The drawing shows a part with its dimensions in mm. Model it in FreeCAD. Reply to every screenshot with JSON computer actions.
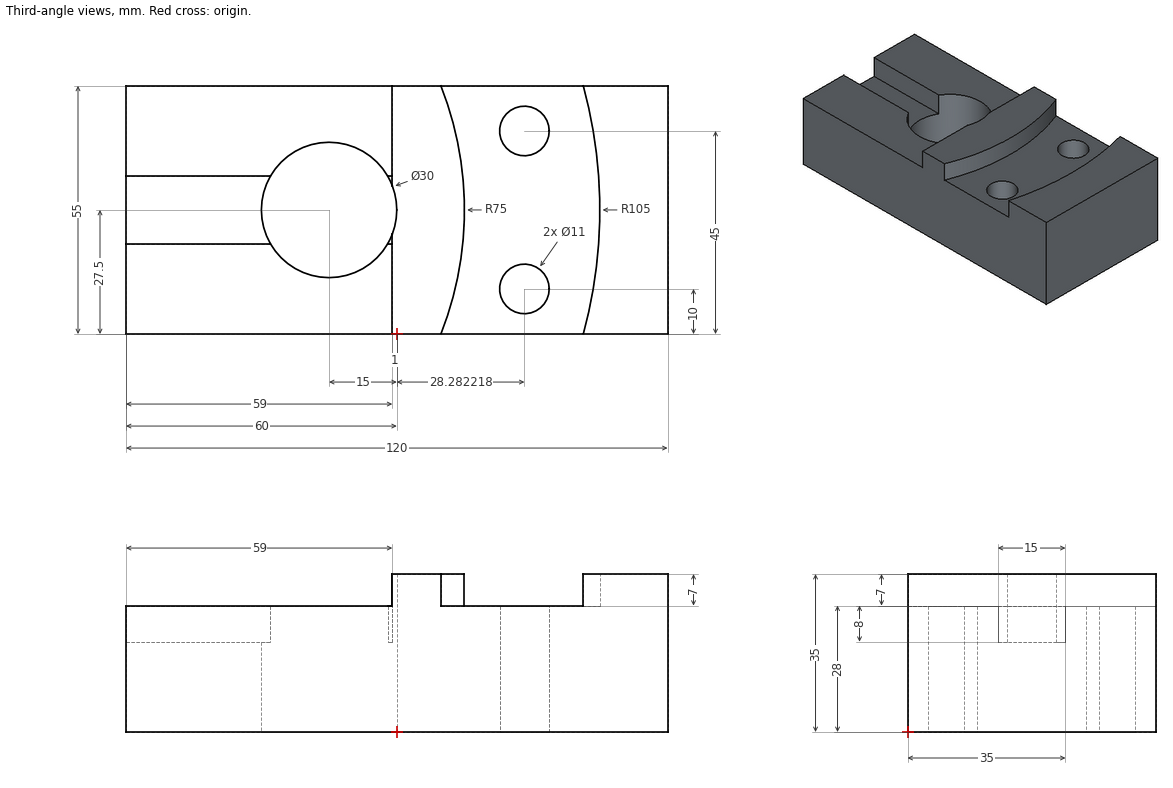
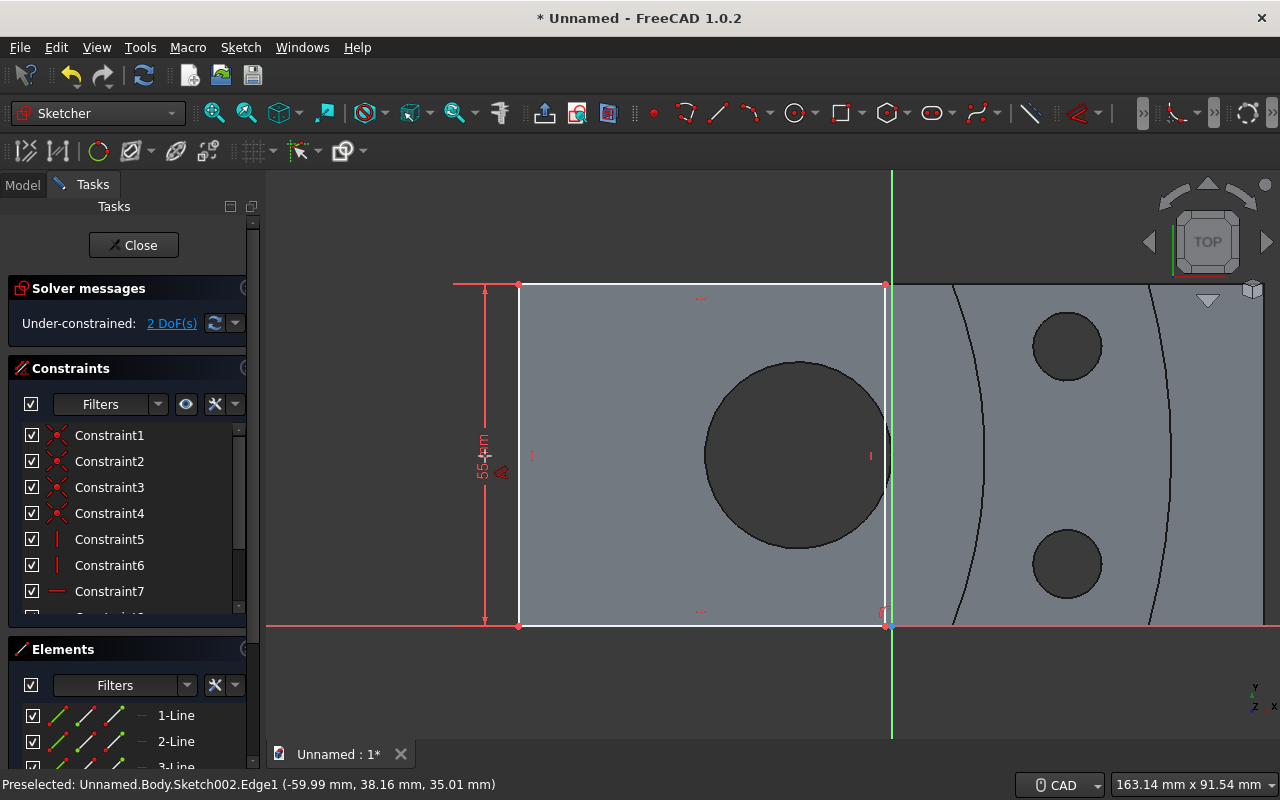
{"action": "left_click", "coordinate": [629, 626]}
{"action": "left_click", "coordinate": [702, 660]}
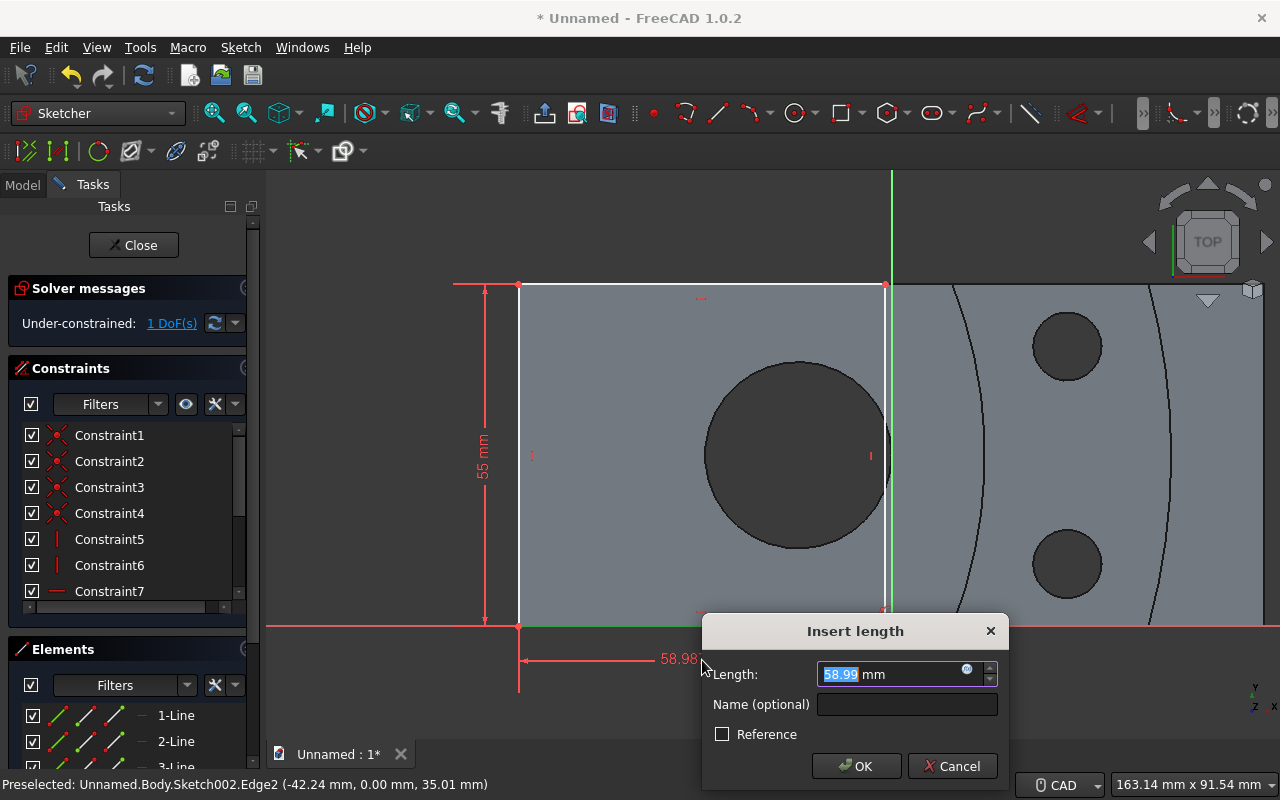
{"action": "type", "text": "59"}
{"action": "key", "text": "Return"}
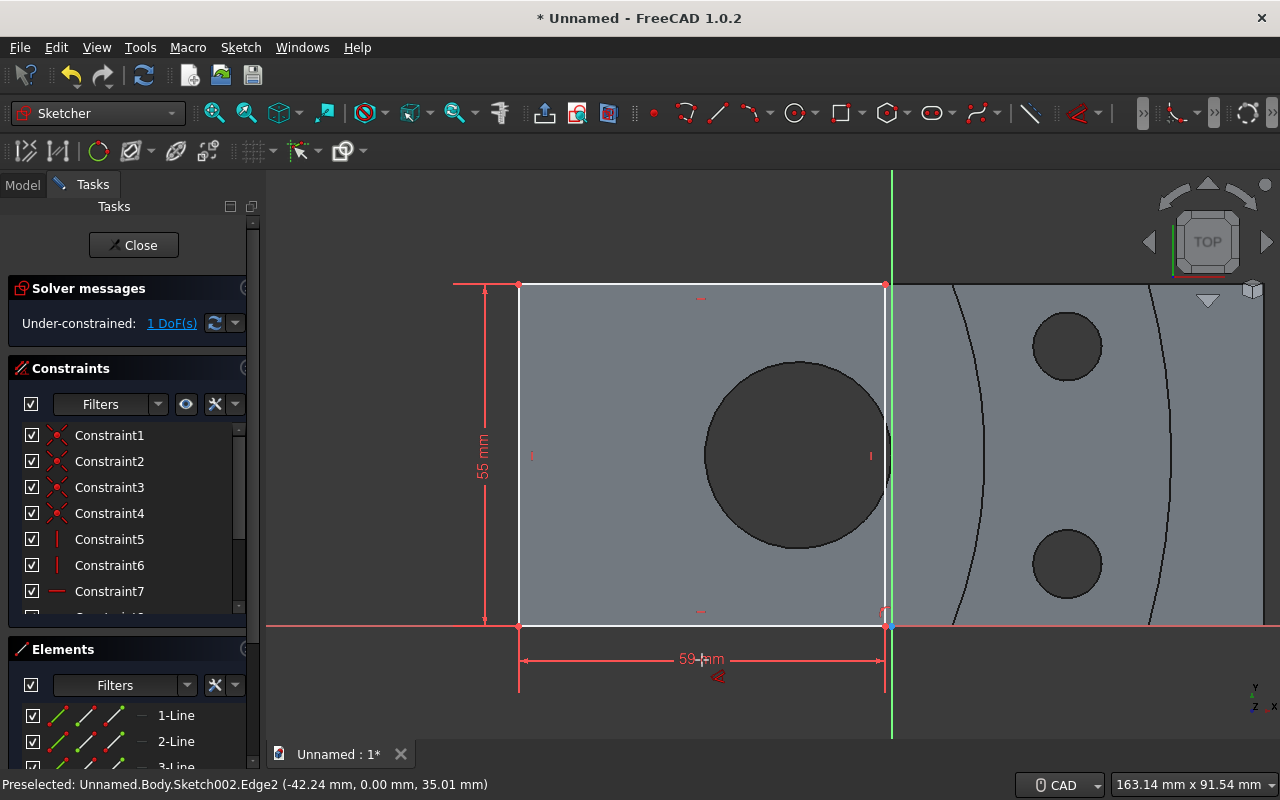
{"action": "scroll", "coordinate": [885, 626], "scroll_direction": "up", "scroll_amount": 10}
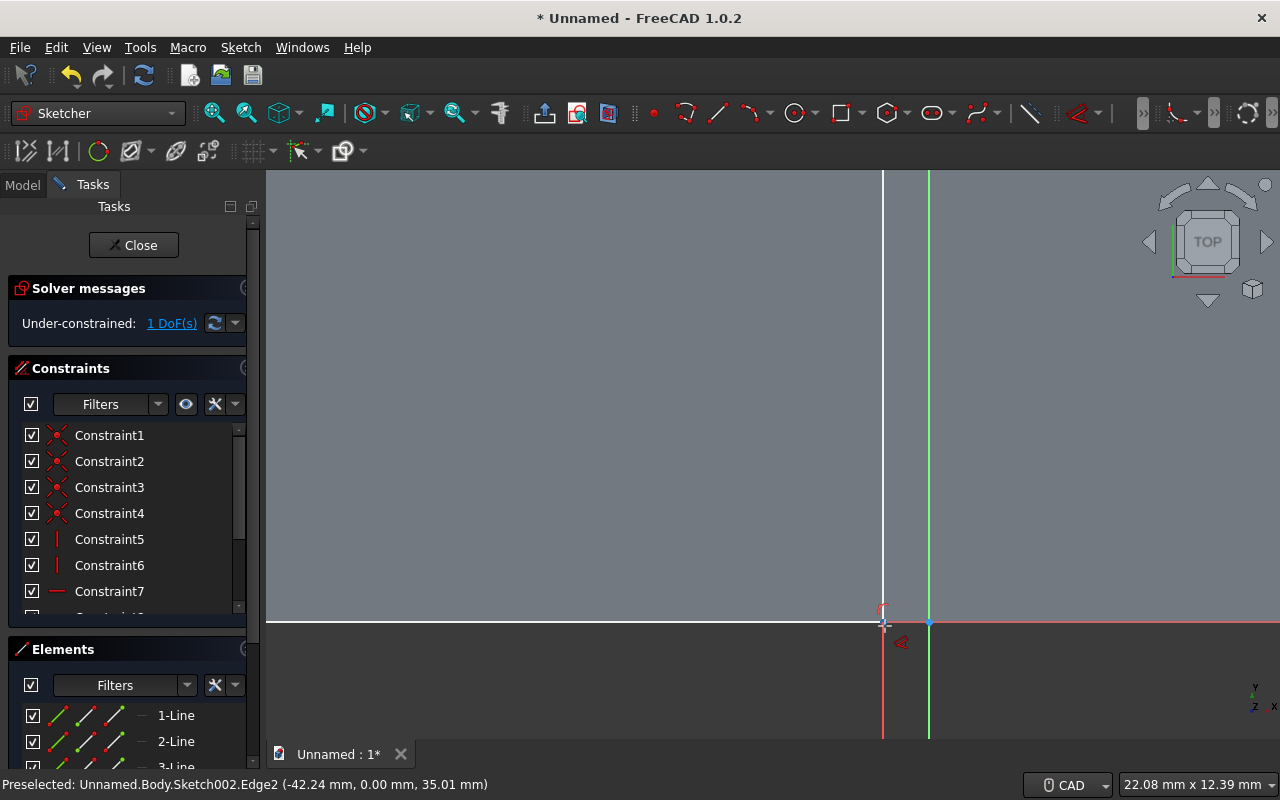
{"action": "left_click", "coordinate": [883, 622]}
{"action": "left_click", "coordinate": [906, 656]}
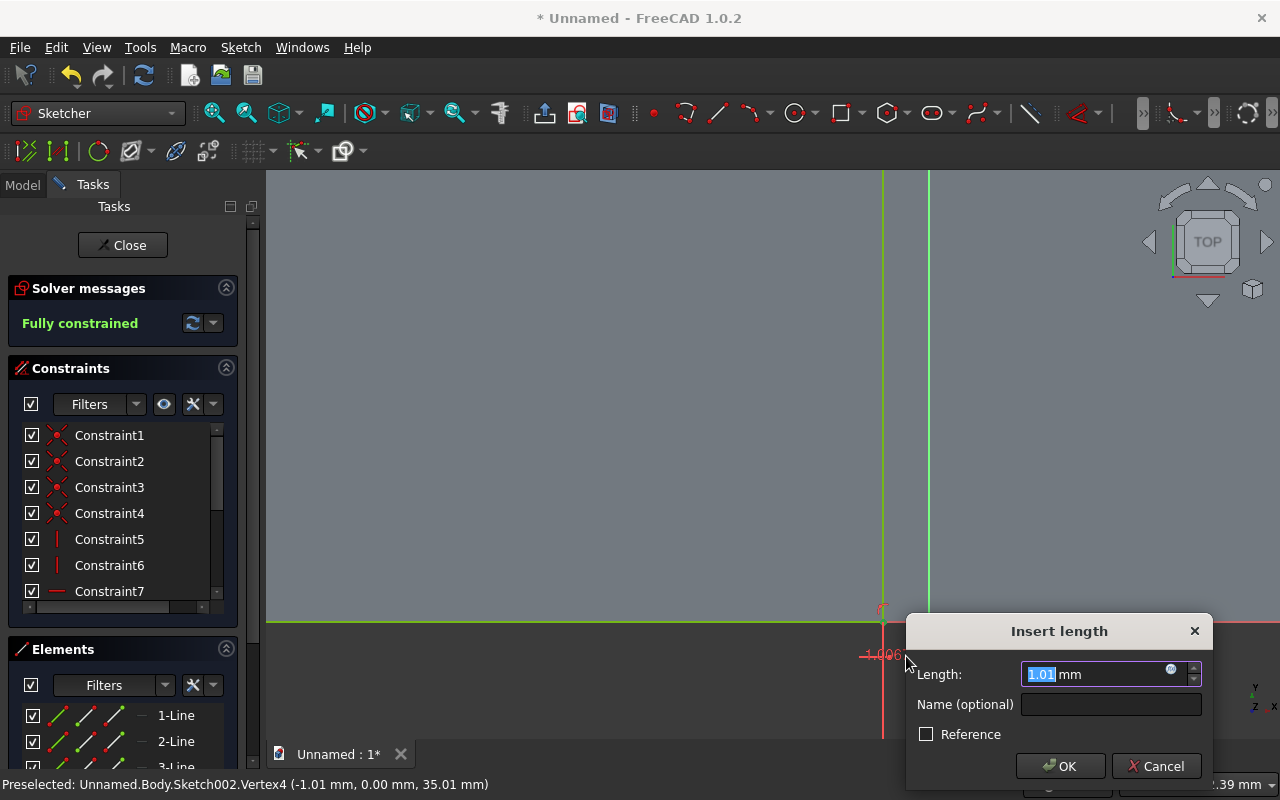
{"action": "type", "text": "1"}
{"action": "key", "text": "Return"}
{"action": "key", "text": "Escape"}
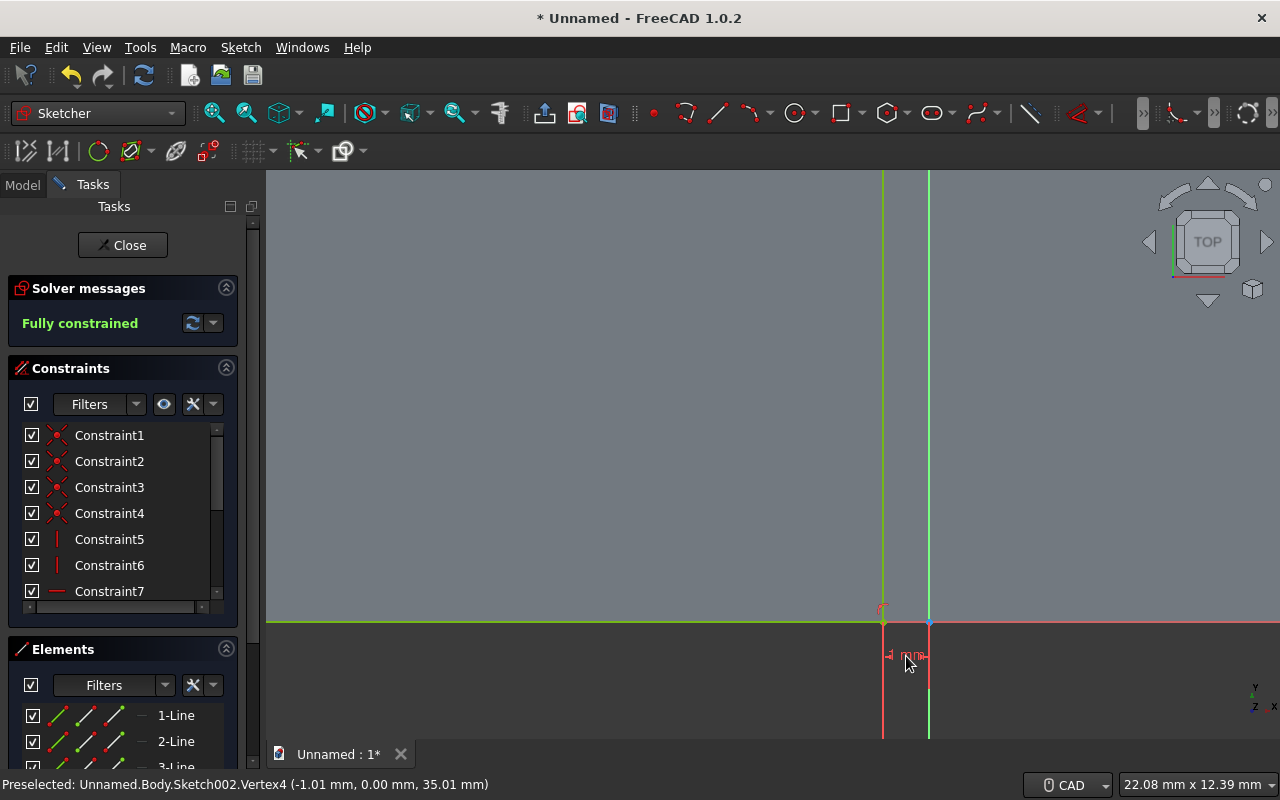
{"action": "left_click", "coordinate": [123, 245]}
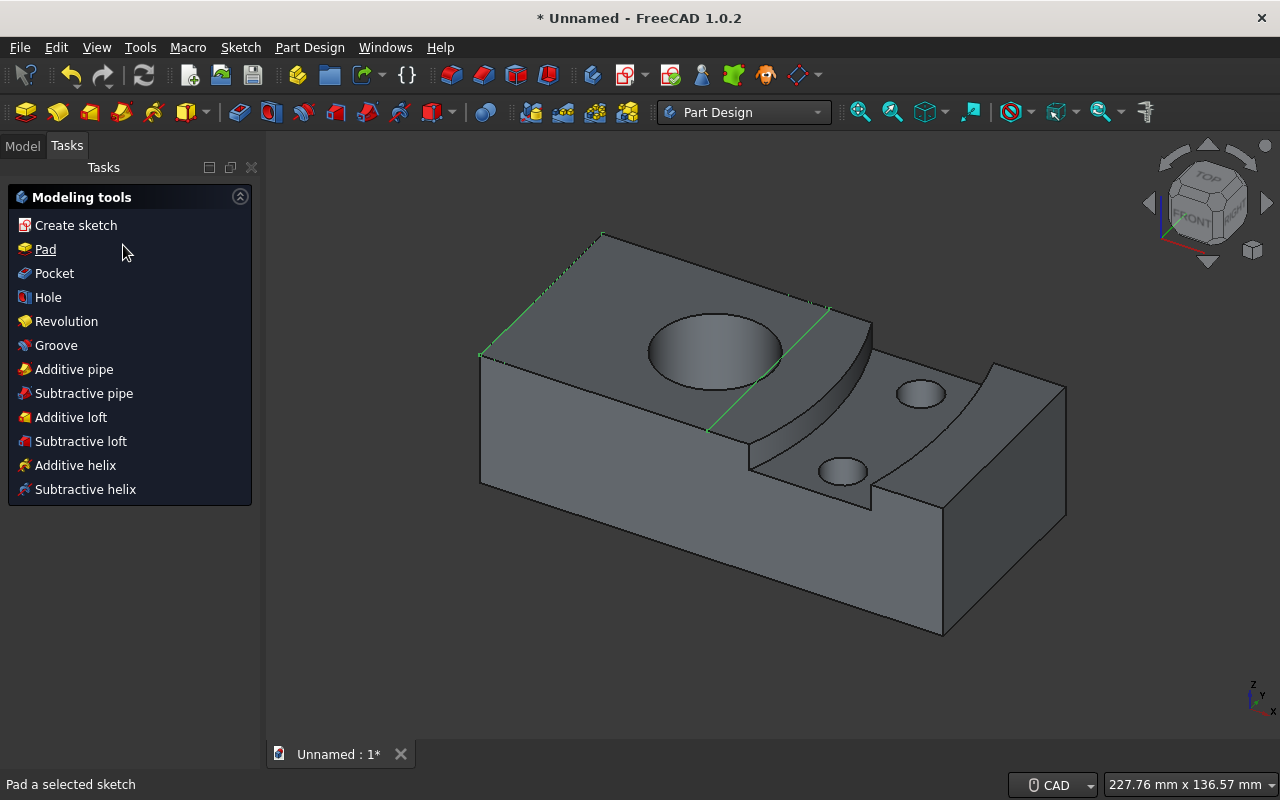
{"action": "left_click", "coordinate": [240, 112]}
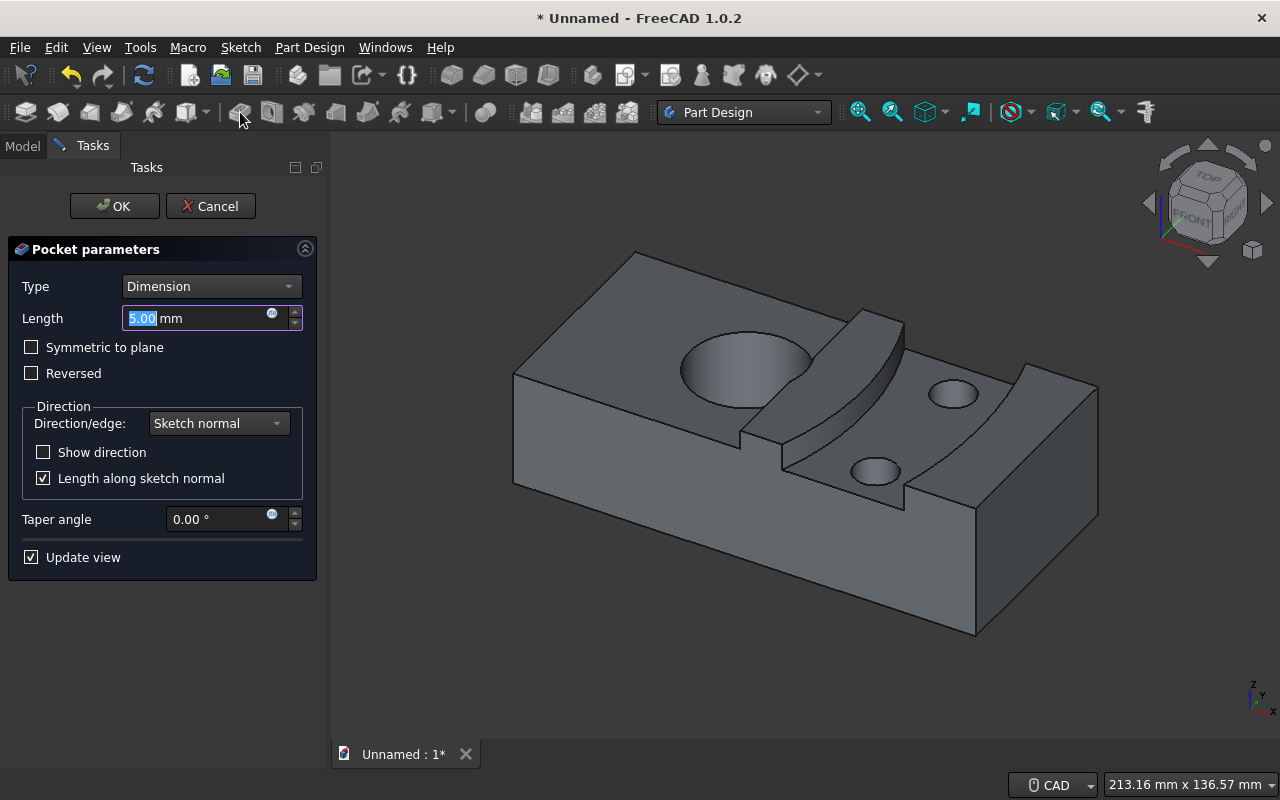
{"action": "type", "text": "7"}
{"action": "key", "text": "Tab"}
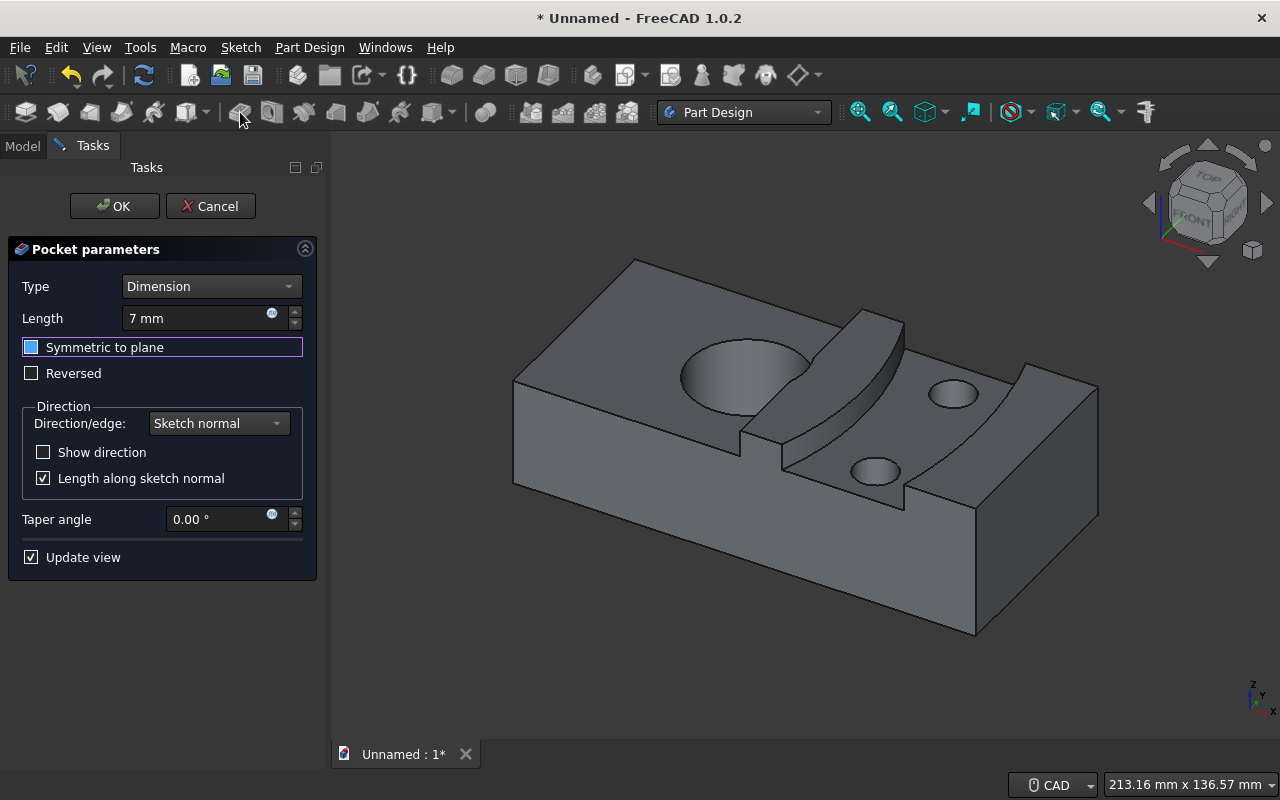
{"action": "left_click", "coordinate": [115, 206]}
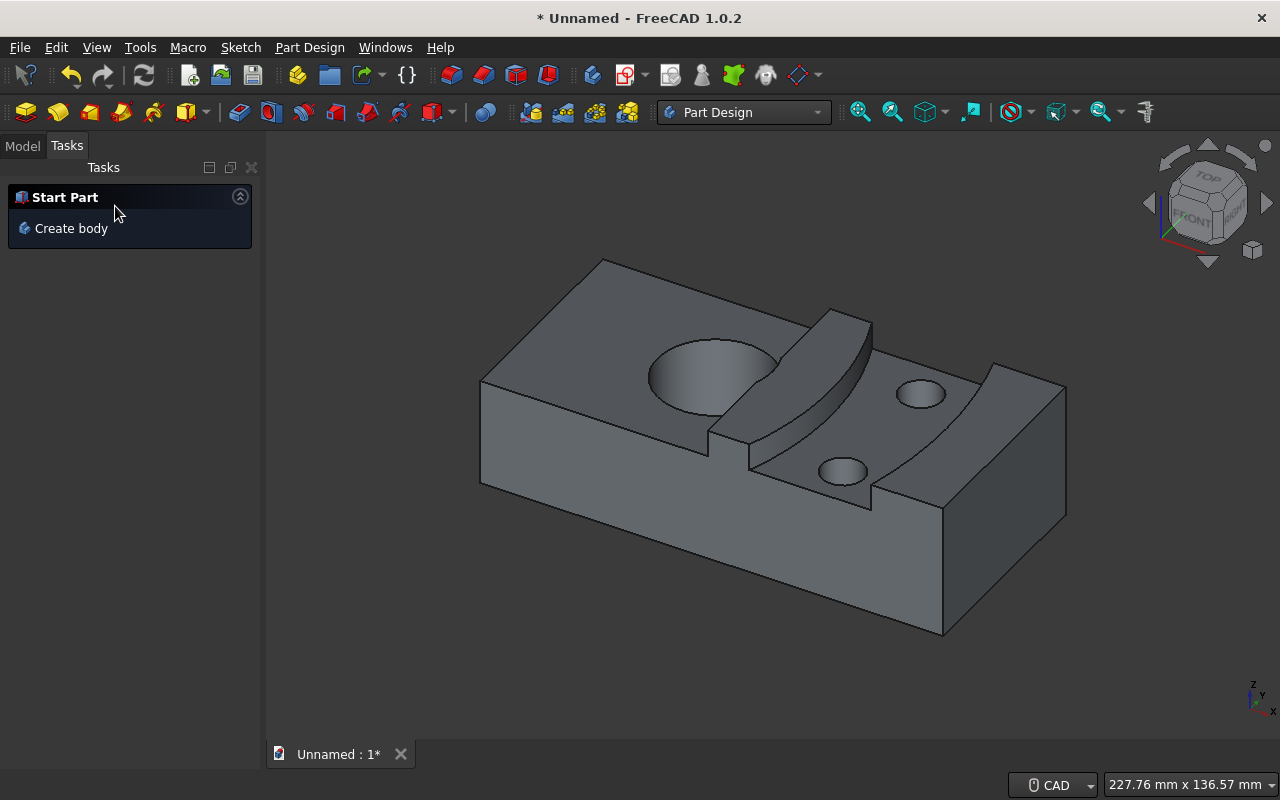
{"action": "key", "text": "6"}